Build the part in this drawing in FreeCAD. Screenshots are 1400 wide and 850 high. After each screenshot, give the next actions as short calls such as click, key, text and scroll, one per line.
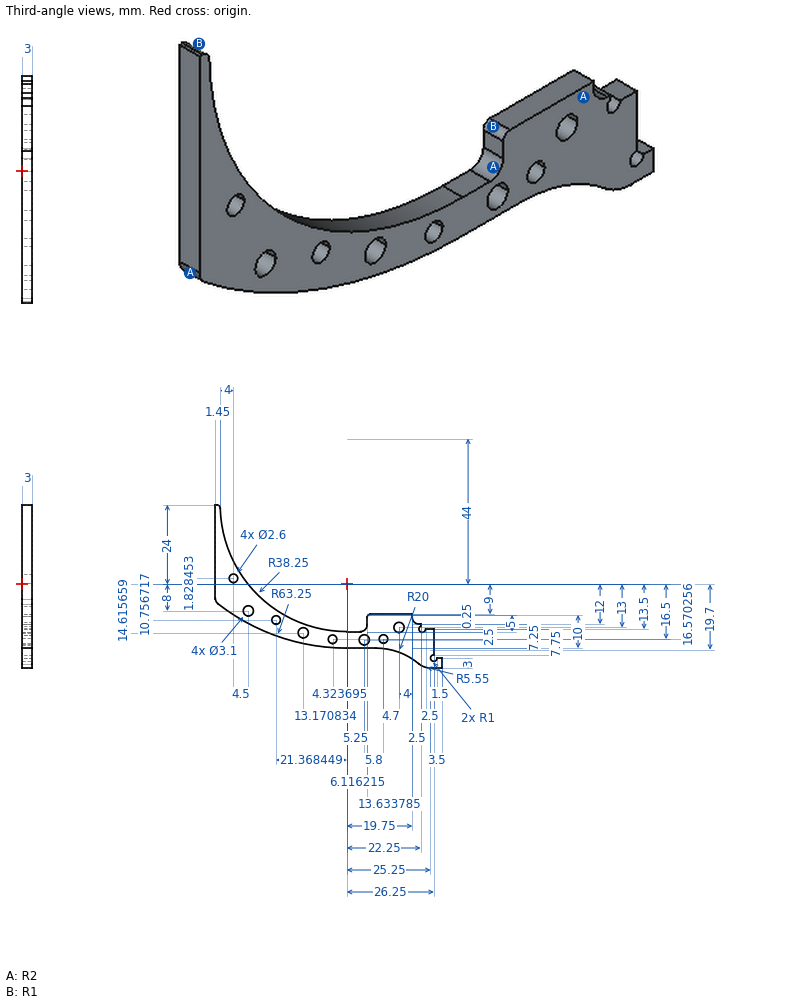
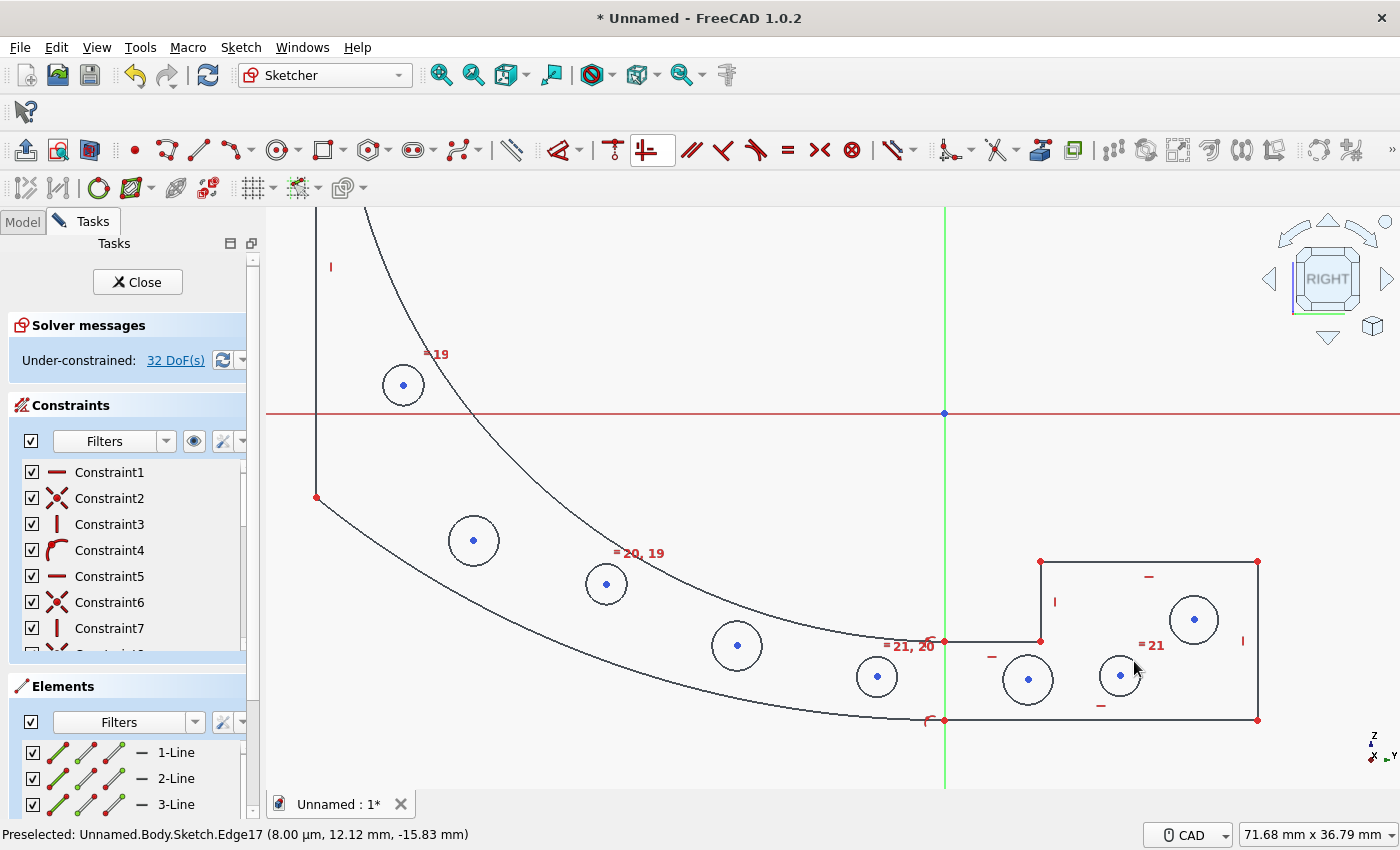
click(491, 523)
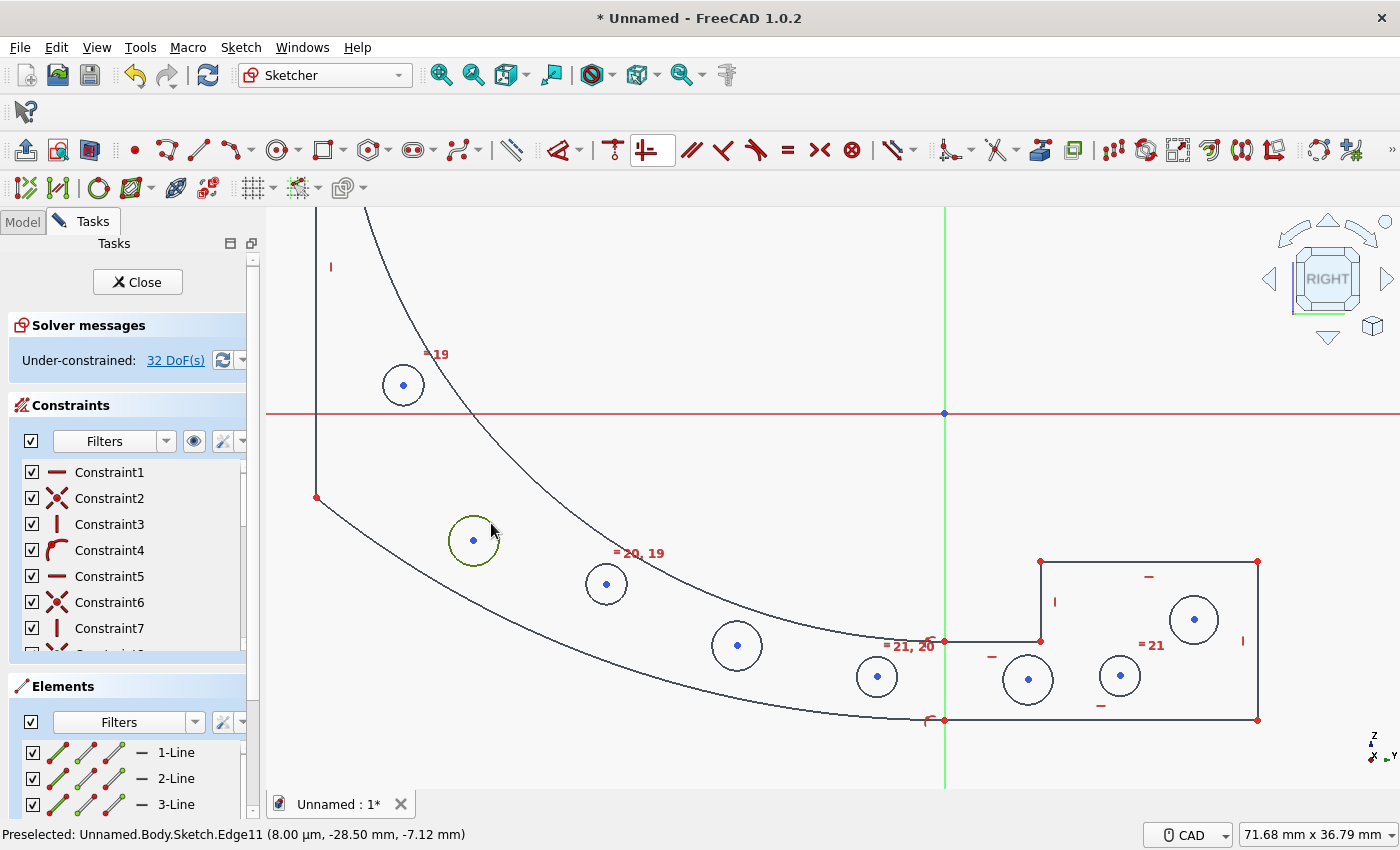
click(754, 628)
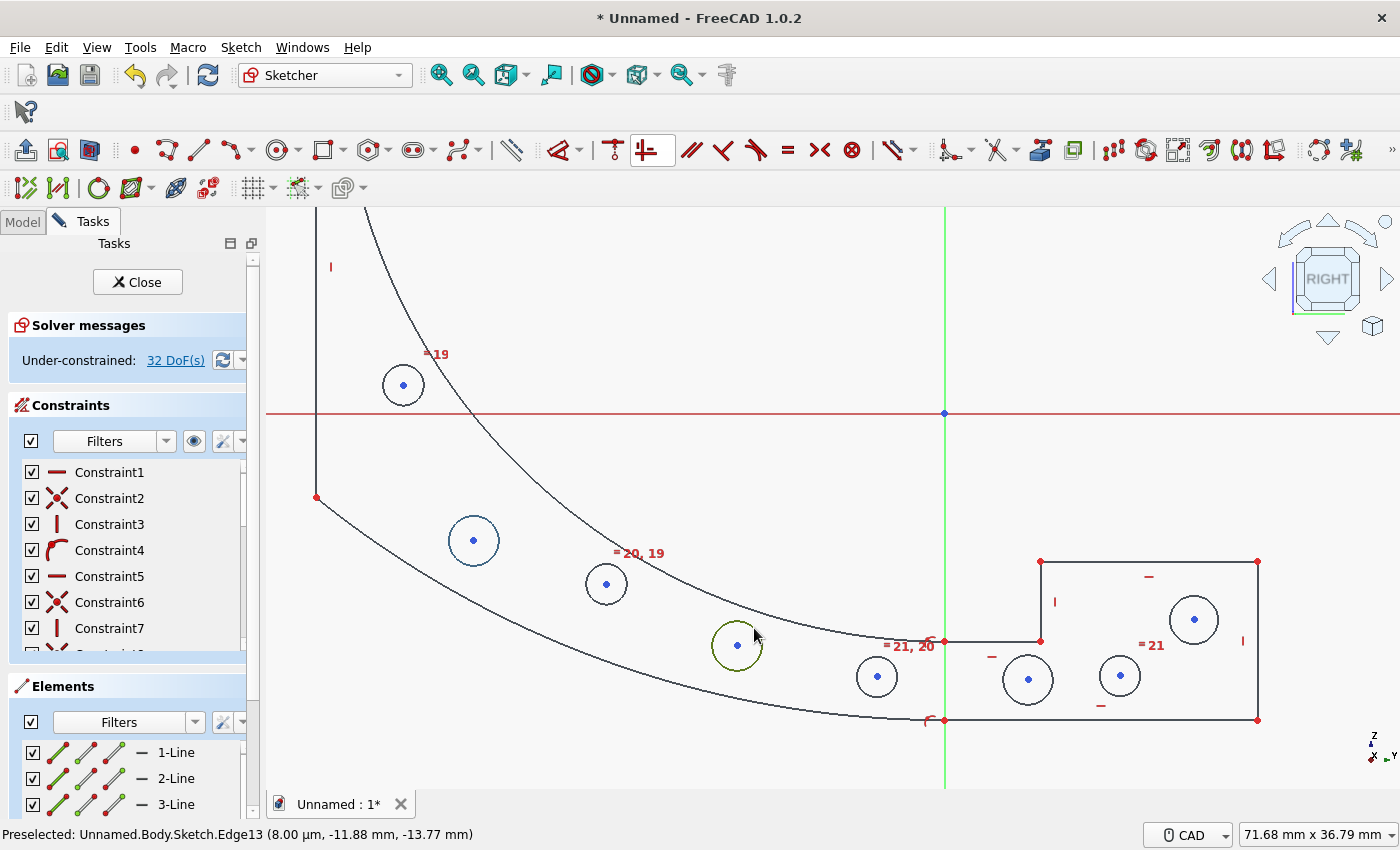
click(1045, 662)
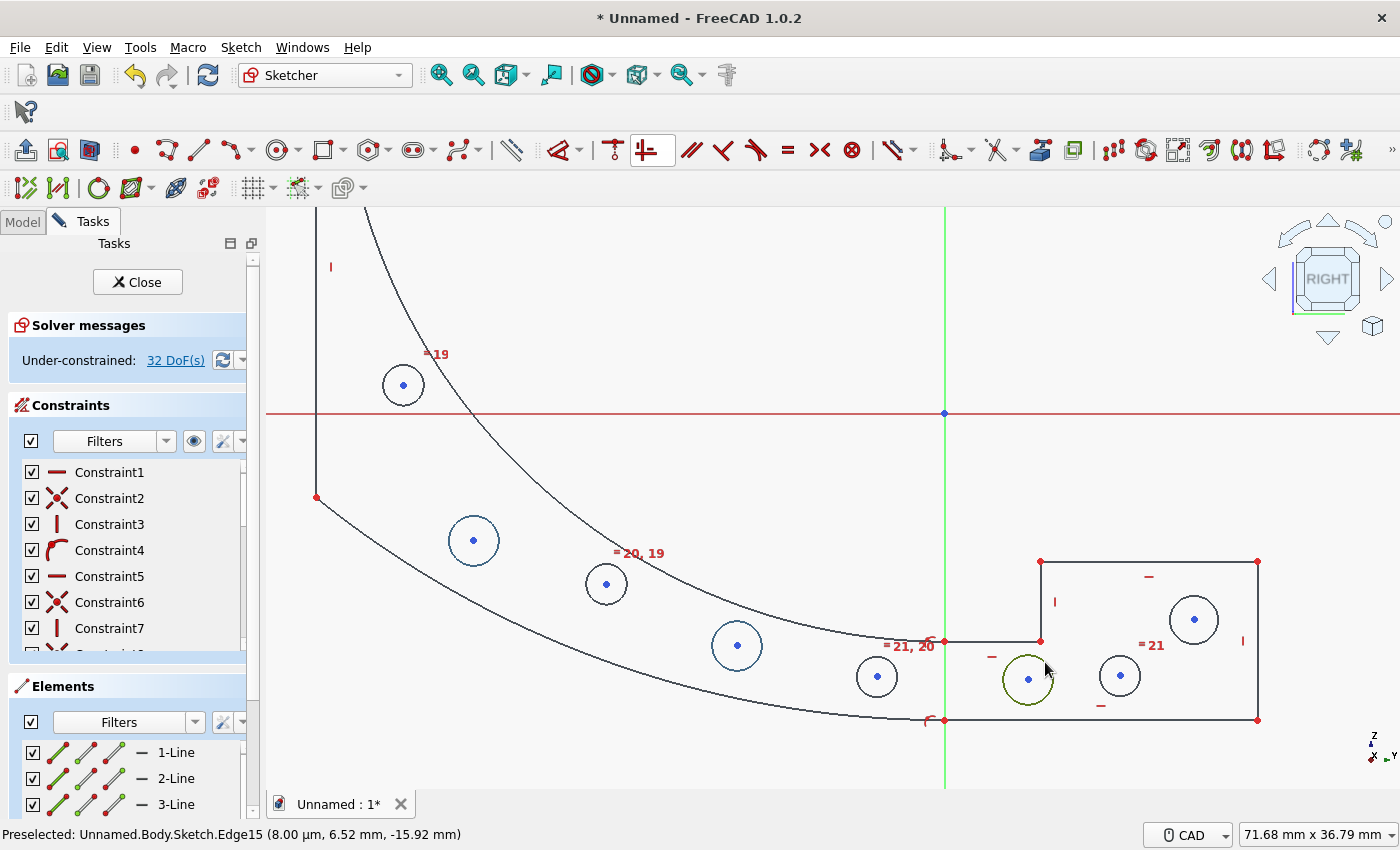
click(1211, 603)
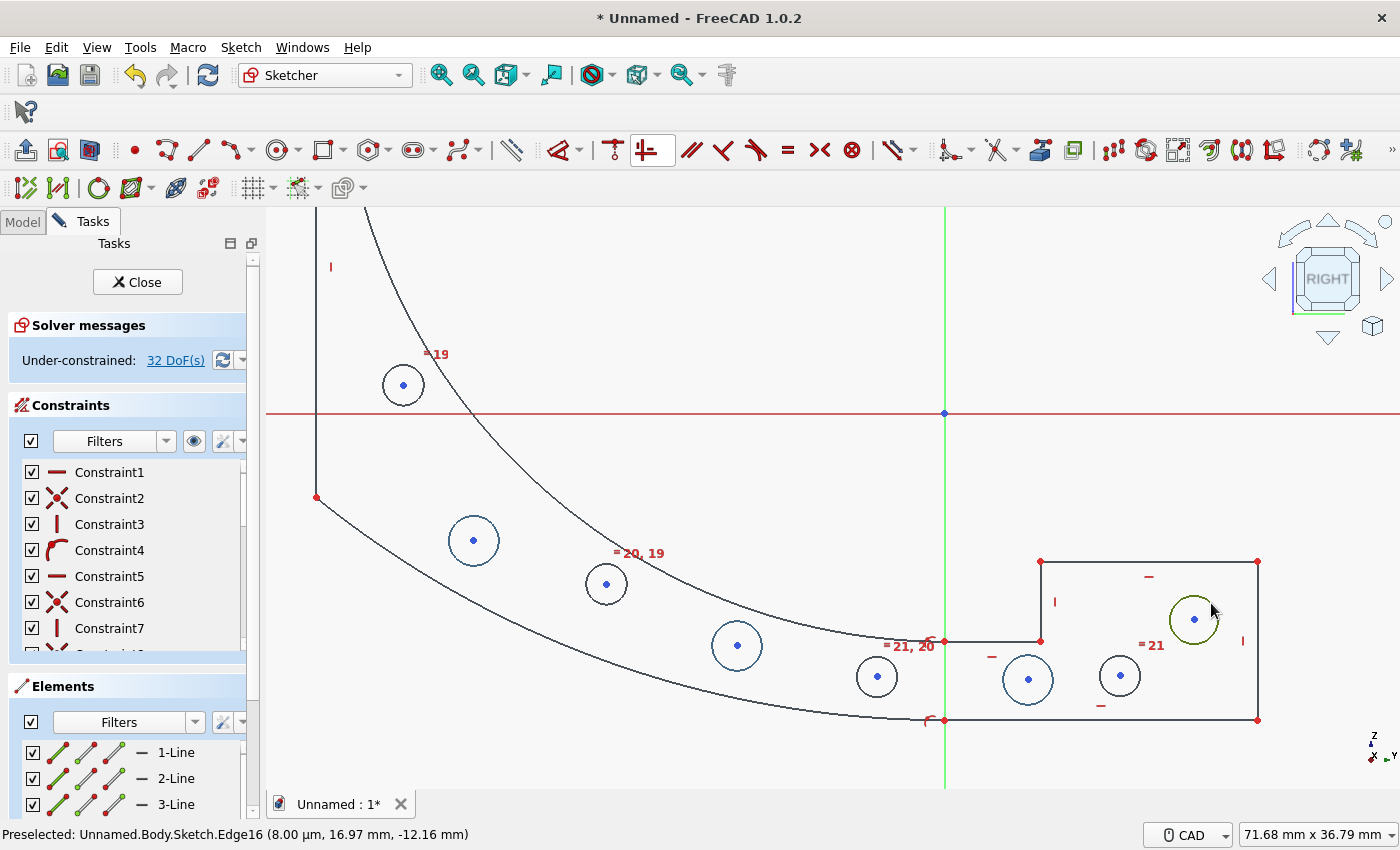
key(e)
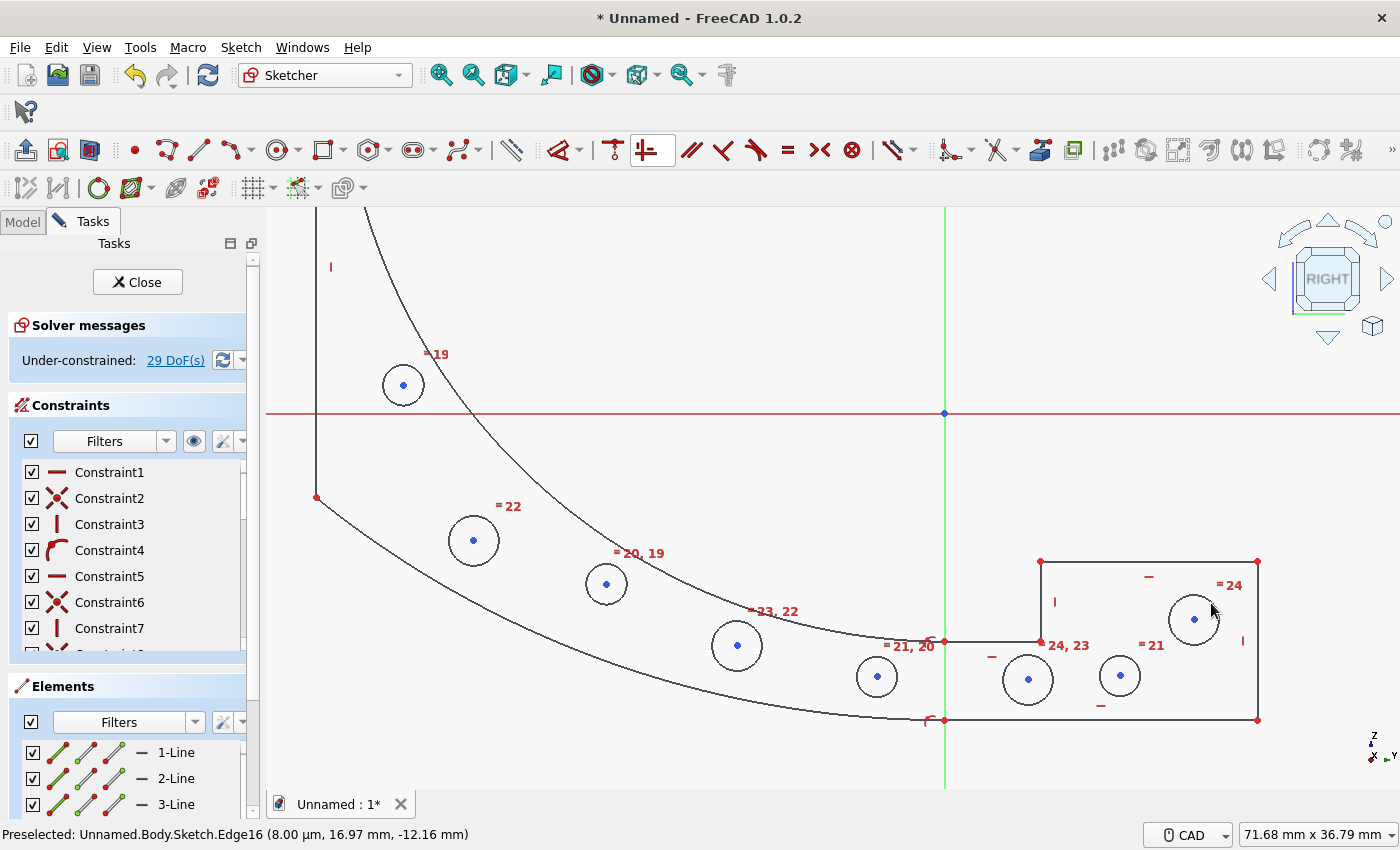
scroll(737, 646, down, 3)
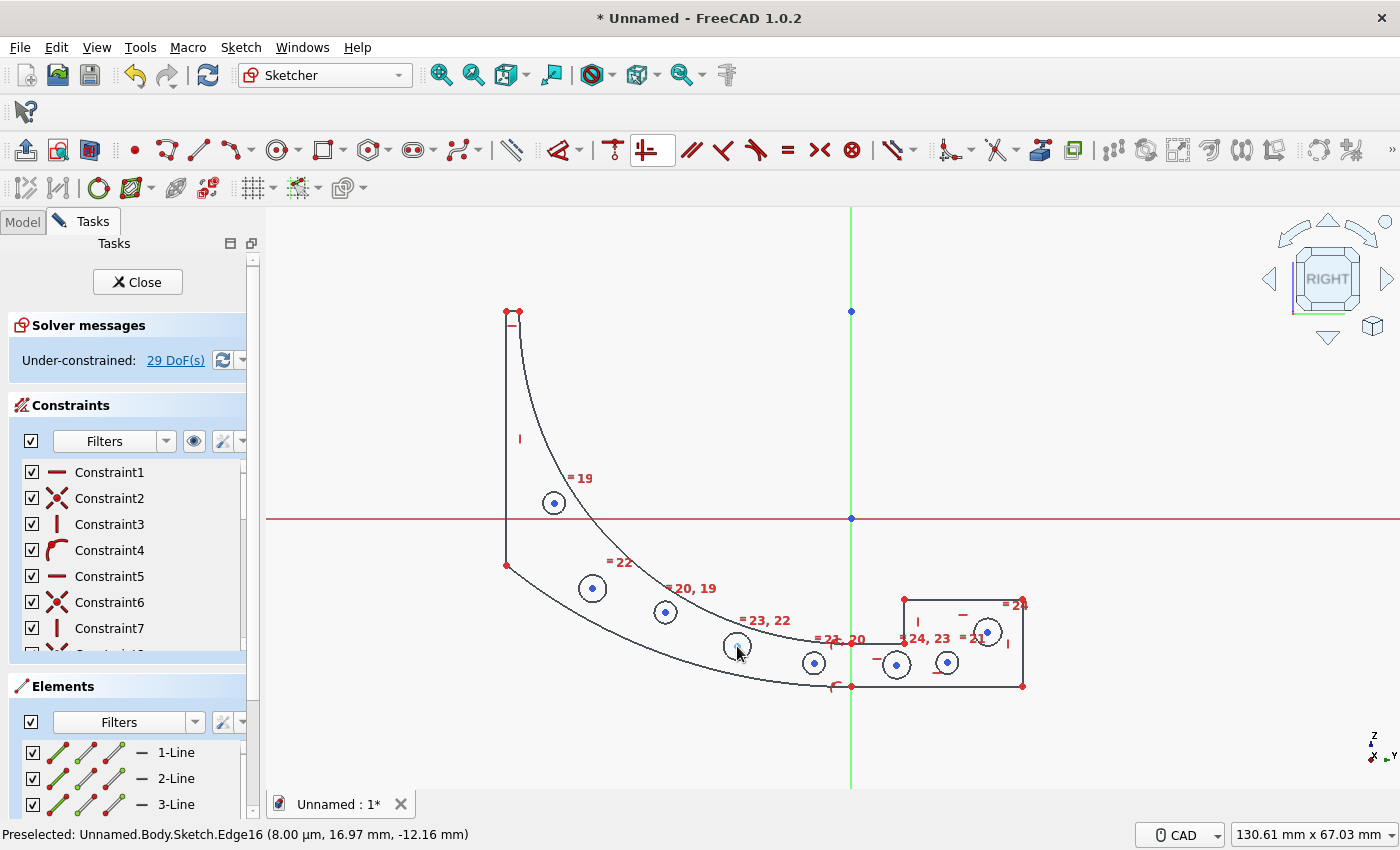
scroll(764, 670, down, 2)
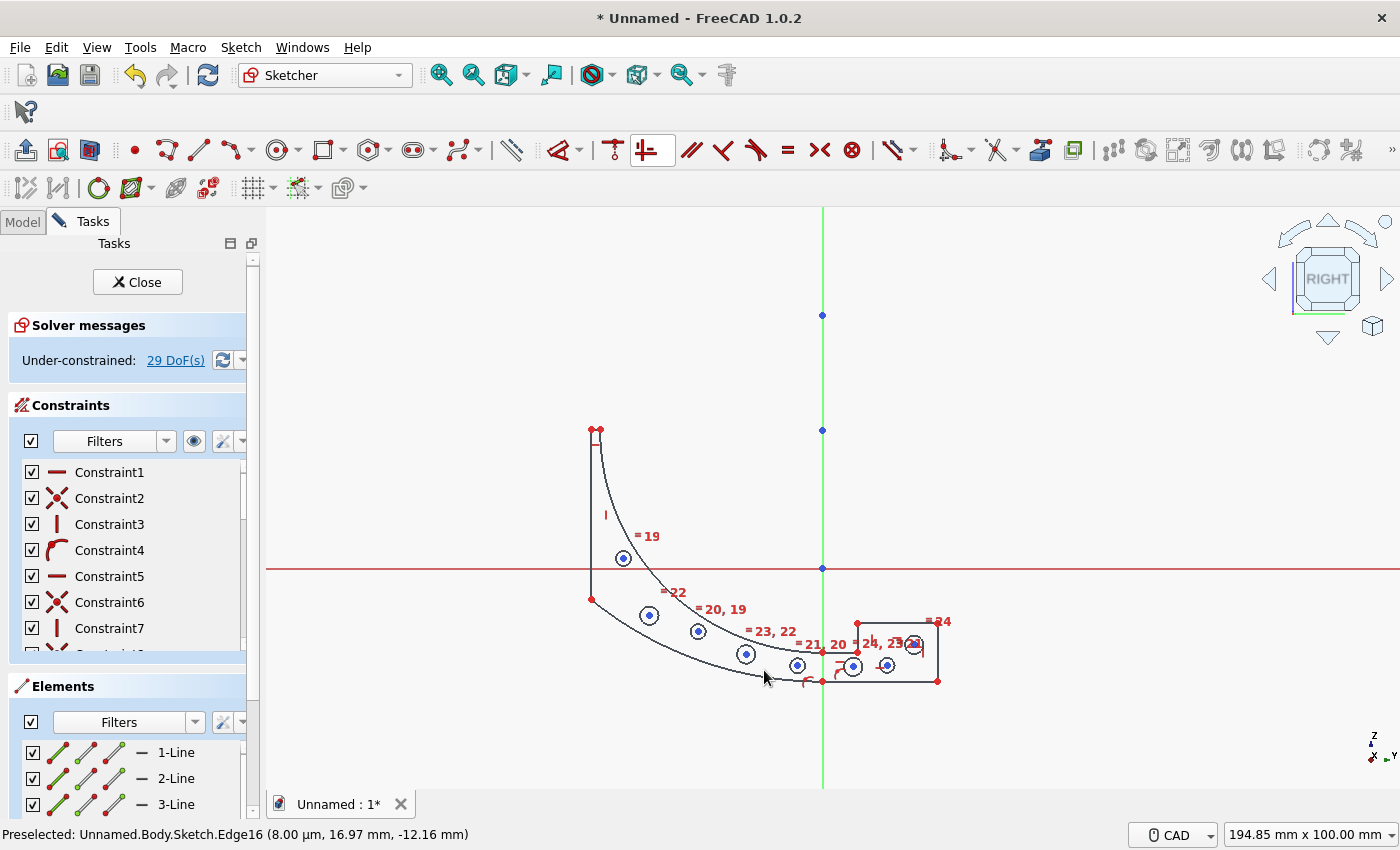
click(822, 315)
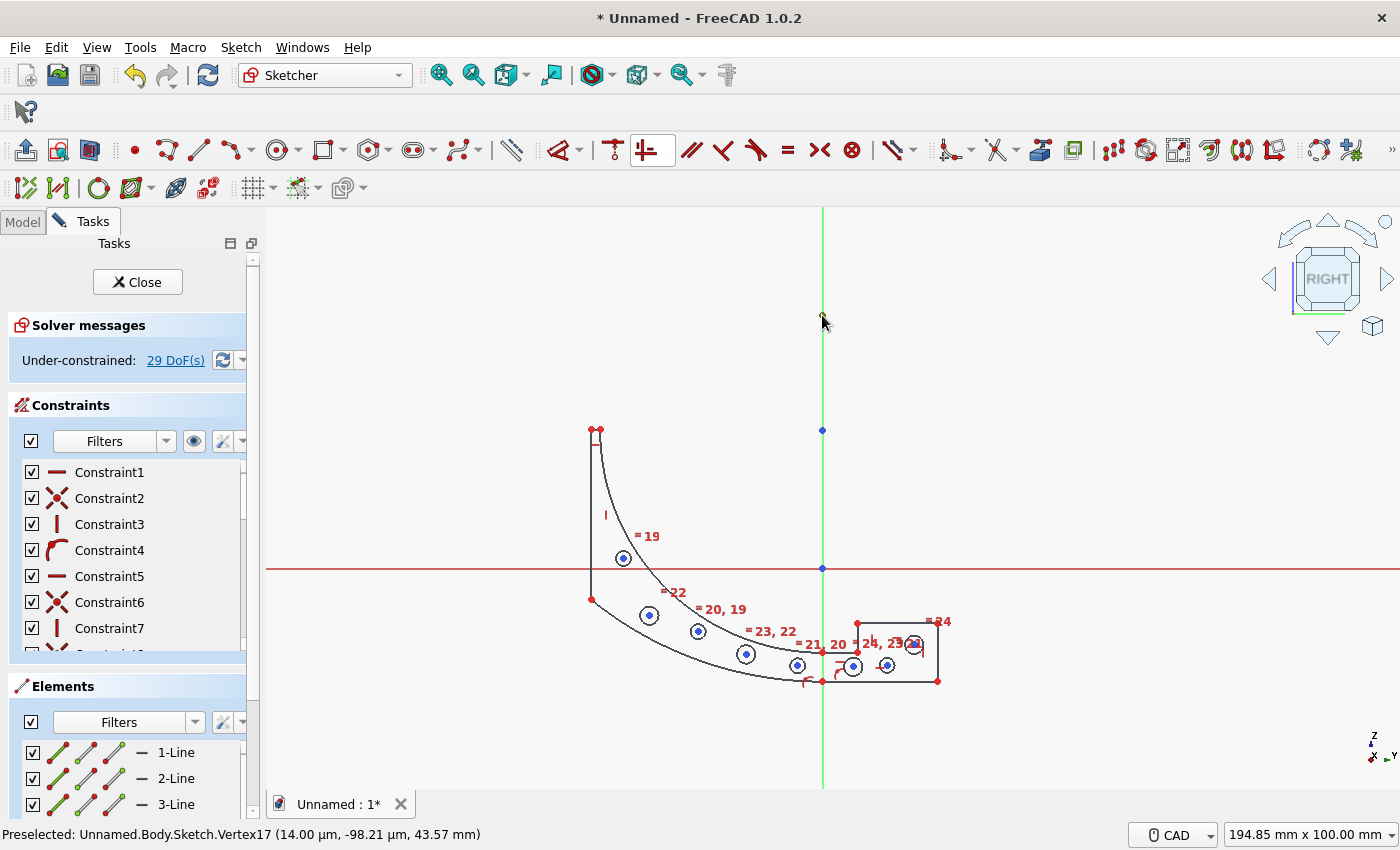
click(823, 723)